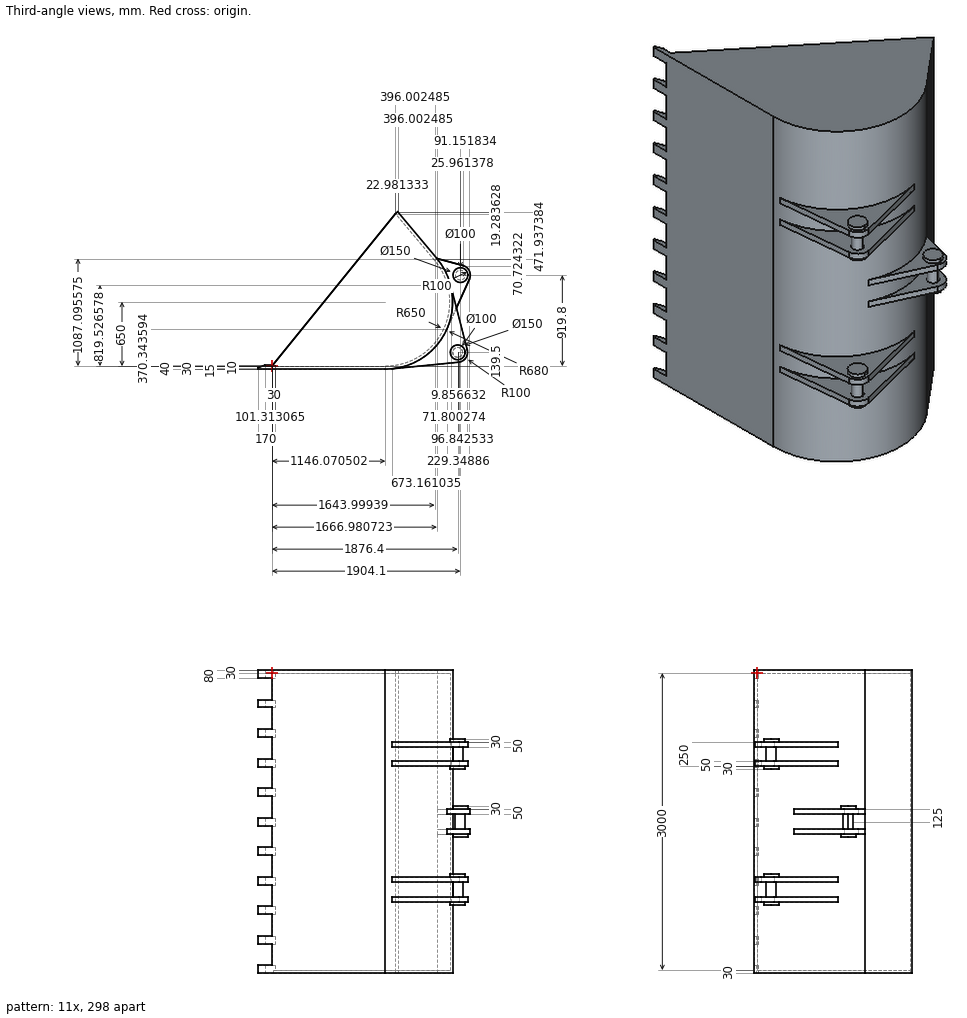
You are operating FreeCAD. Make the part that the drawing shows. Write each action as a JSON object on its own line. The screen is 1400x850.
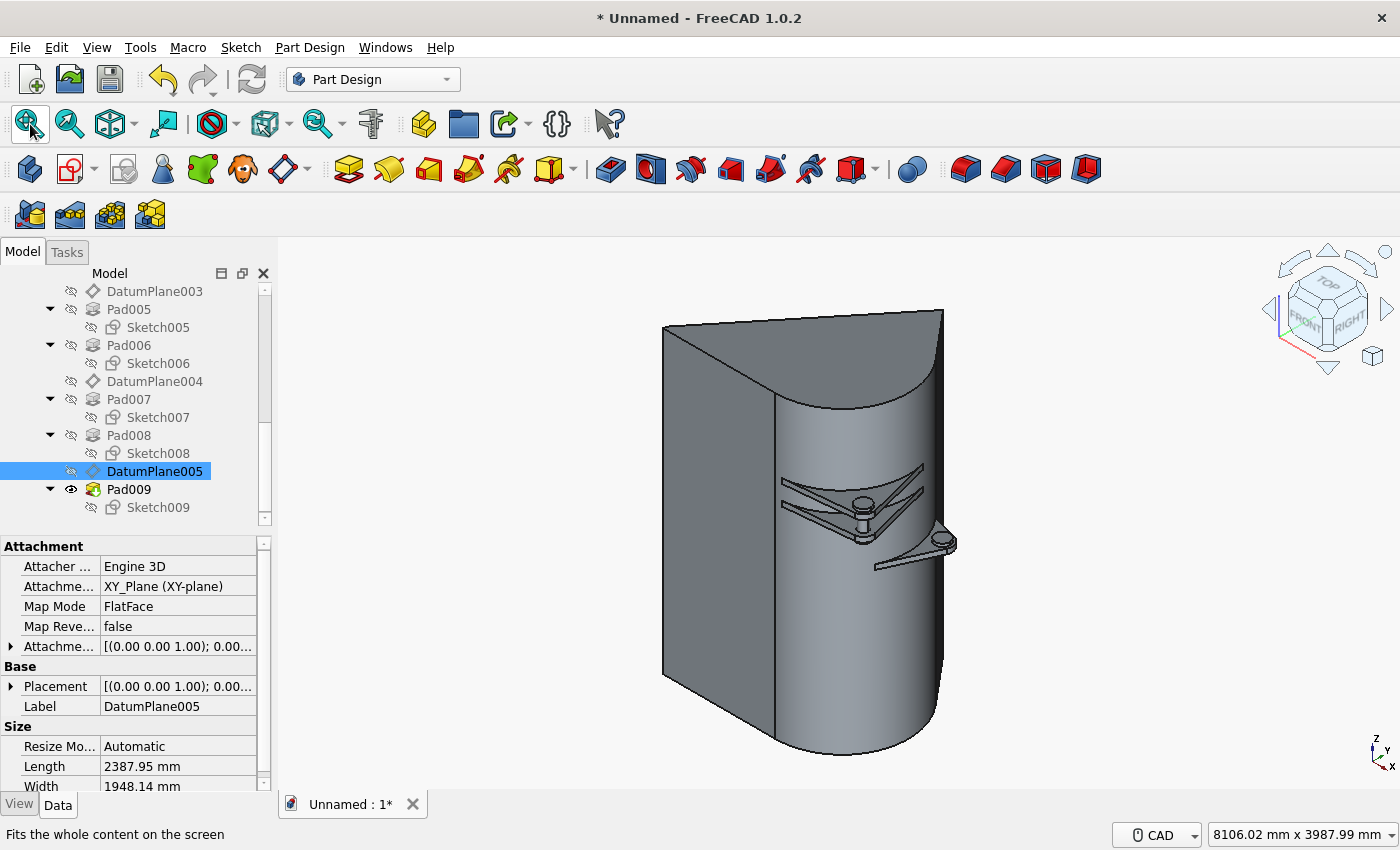
{"action": "scroll", "coordinate": [922, 550], "scroll_direction": "up", "scroll_amount": 4}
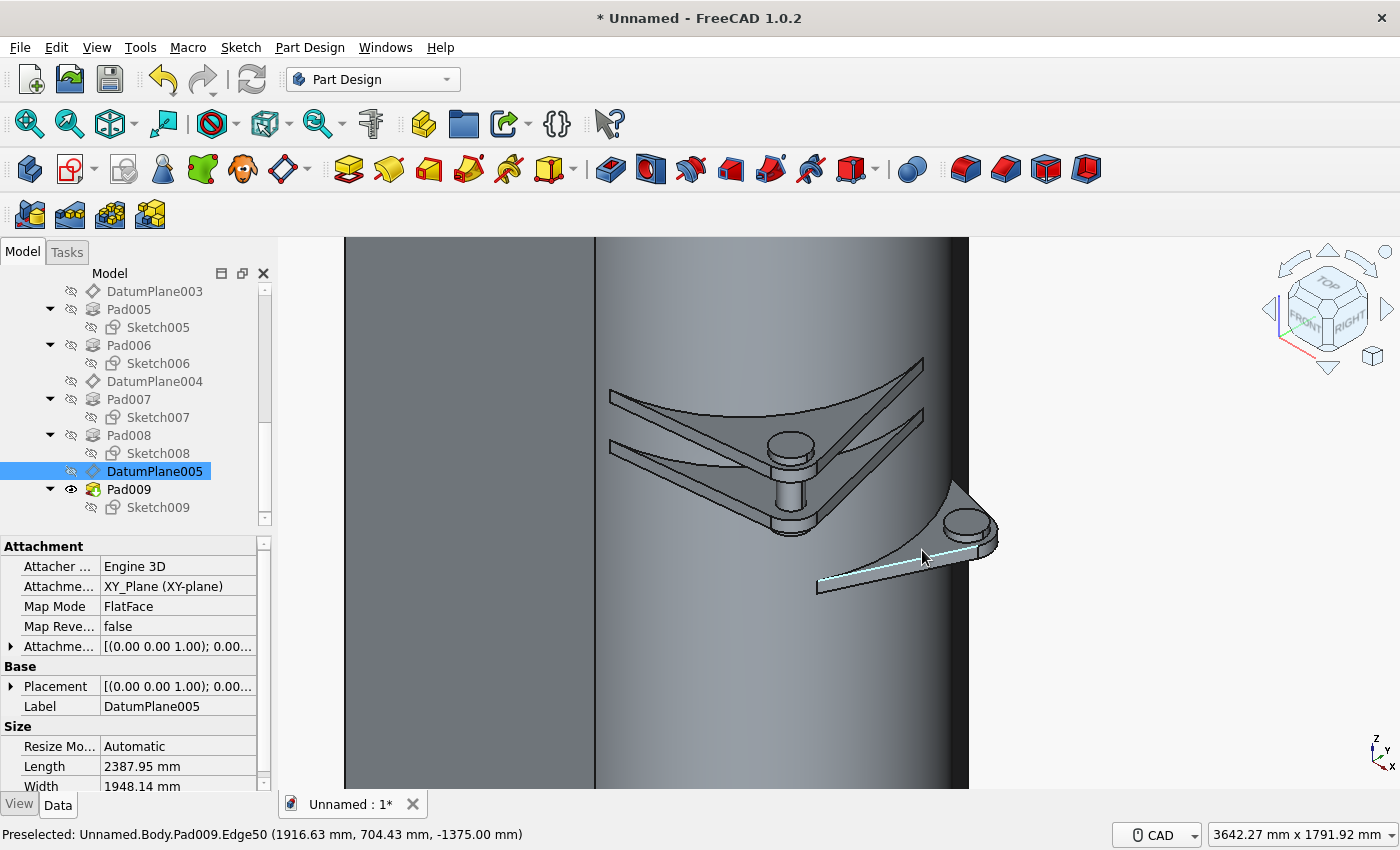
{"action": "left_click", "coordinate": [933, 531]}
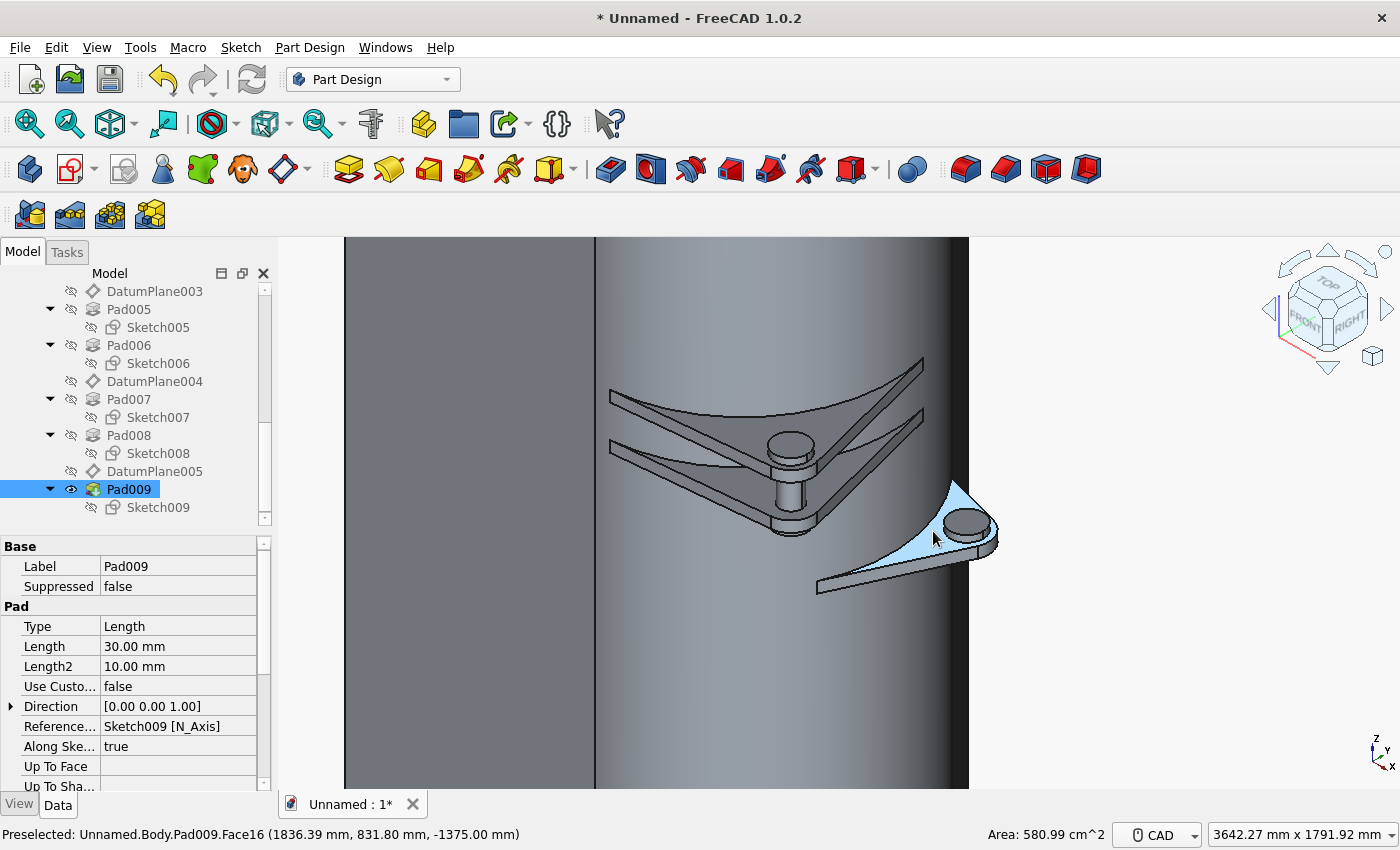
{"action": "left_click", "coordinate": [70, 170]}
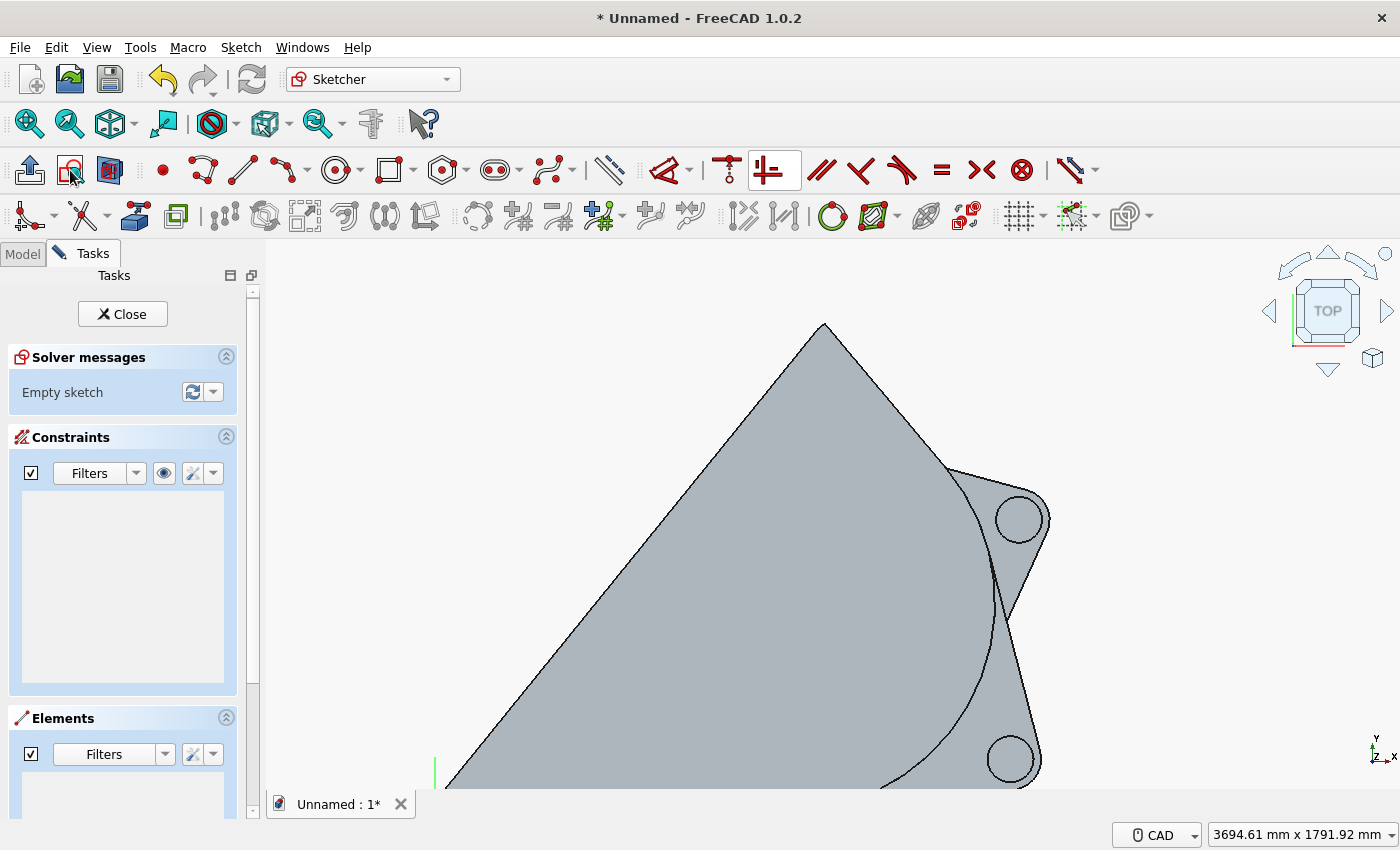
{"action": "scroll", "coordinate": [1044, 520], "scroll_direction": "up", "scroll_amount": 12}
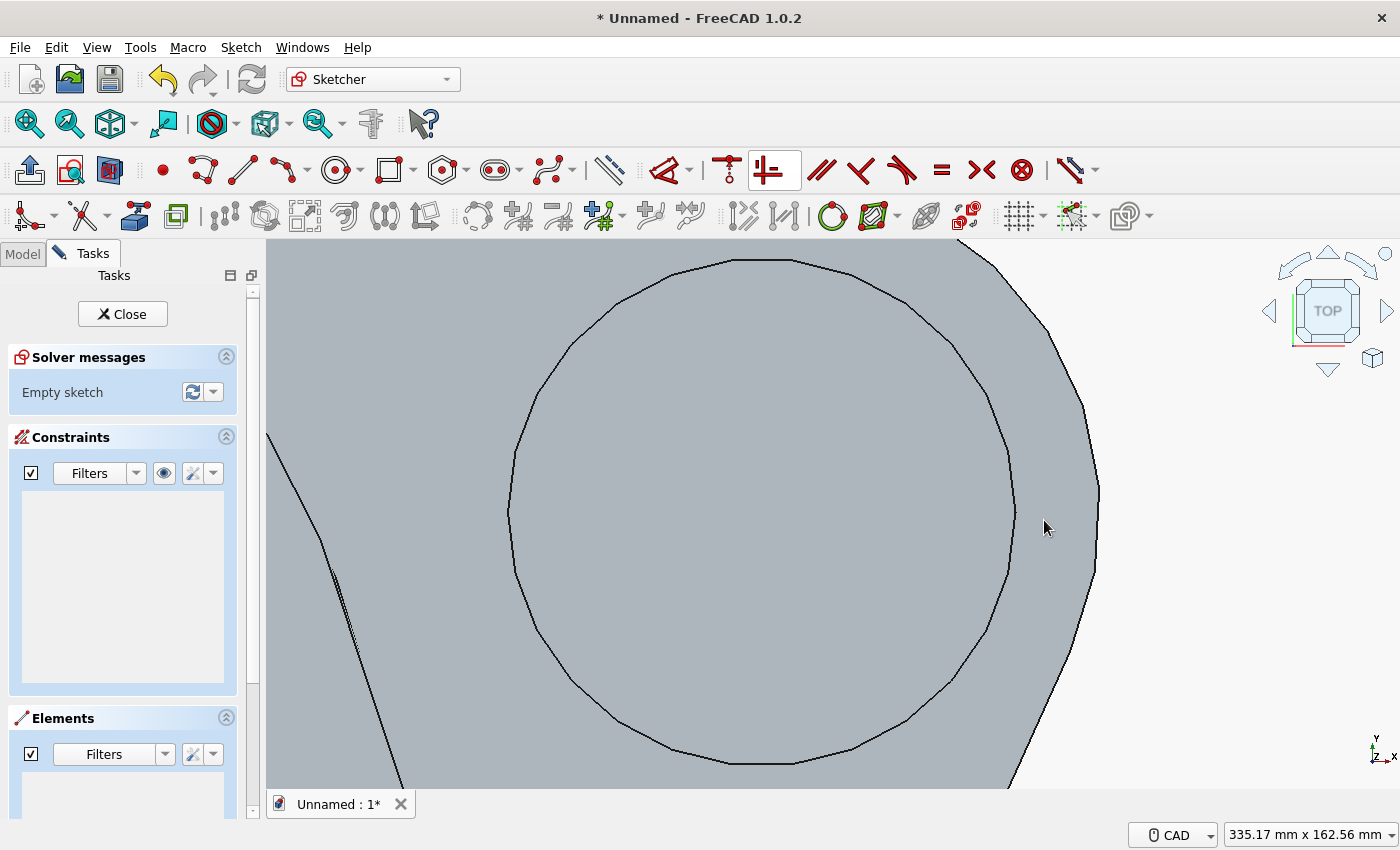
{"action": "left_click", "coordinate": [336, 170]}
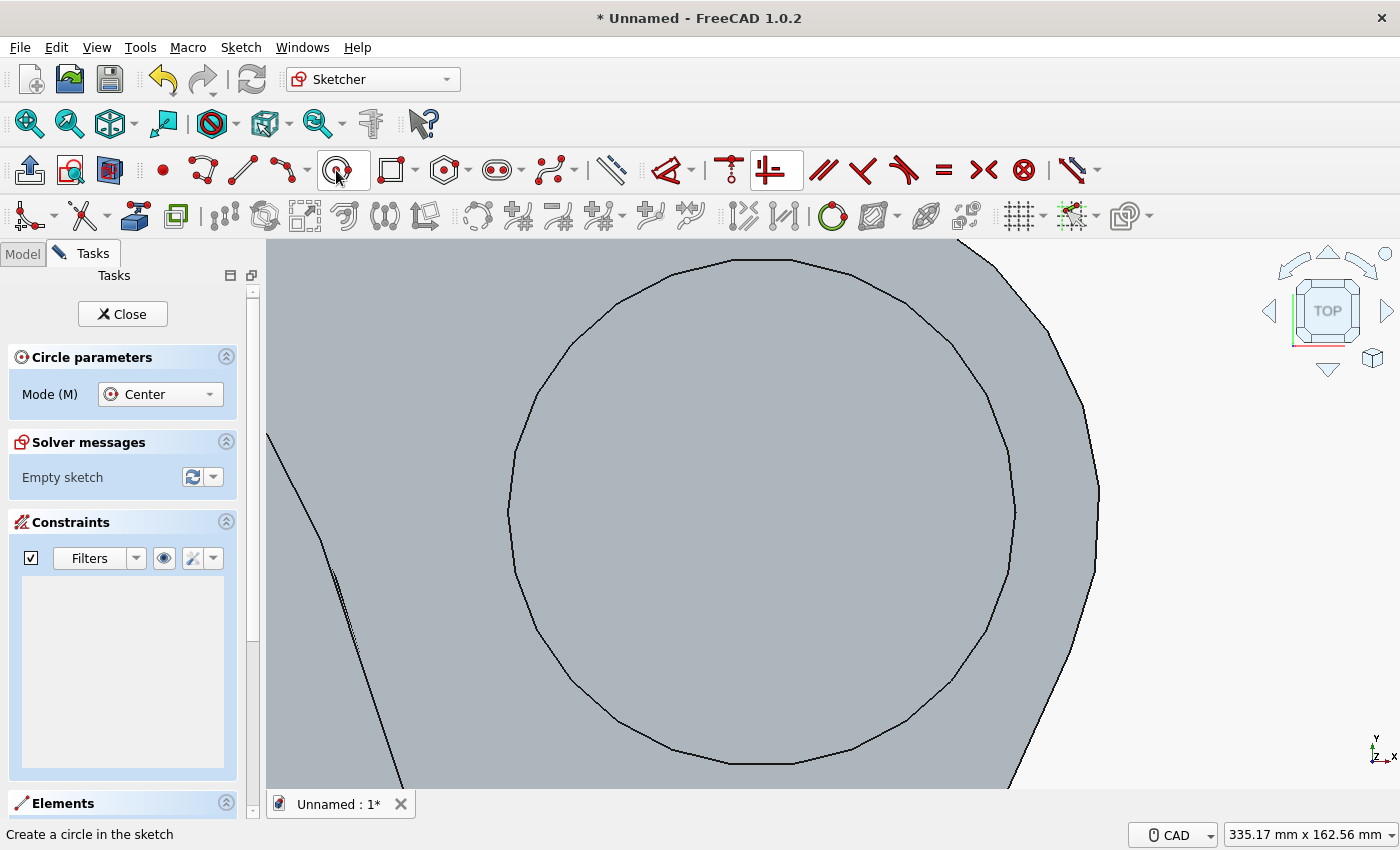
{"action": "left_click", "coordinate": [762, 512]}
{"action": "left_click", "coordinate": [881, 393]}
{"action": "key", "text": "Escape"}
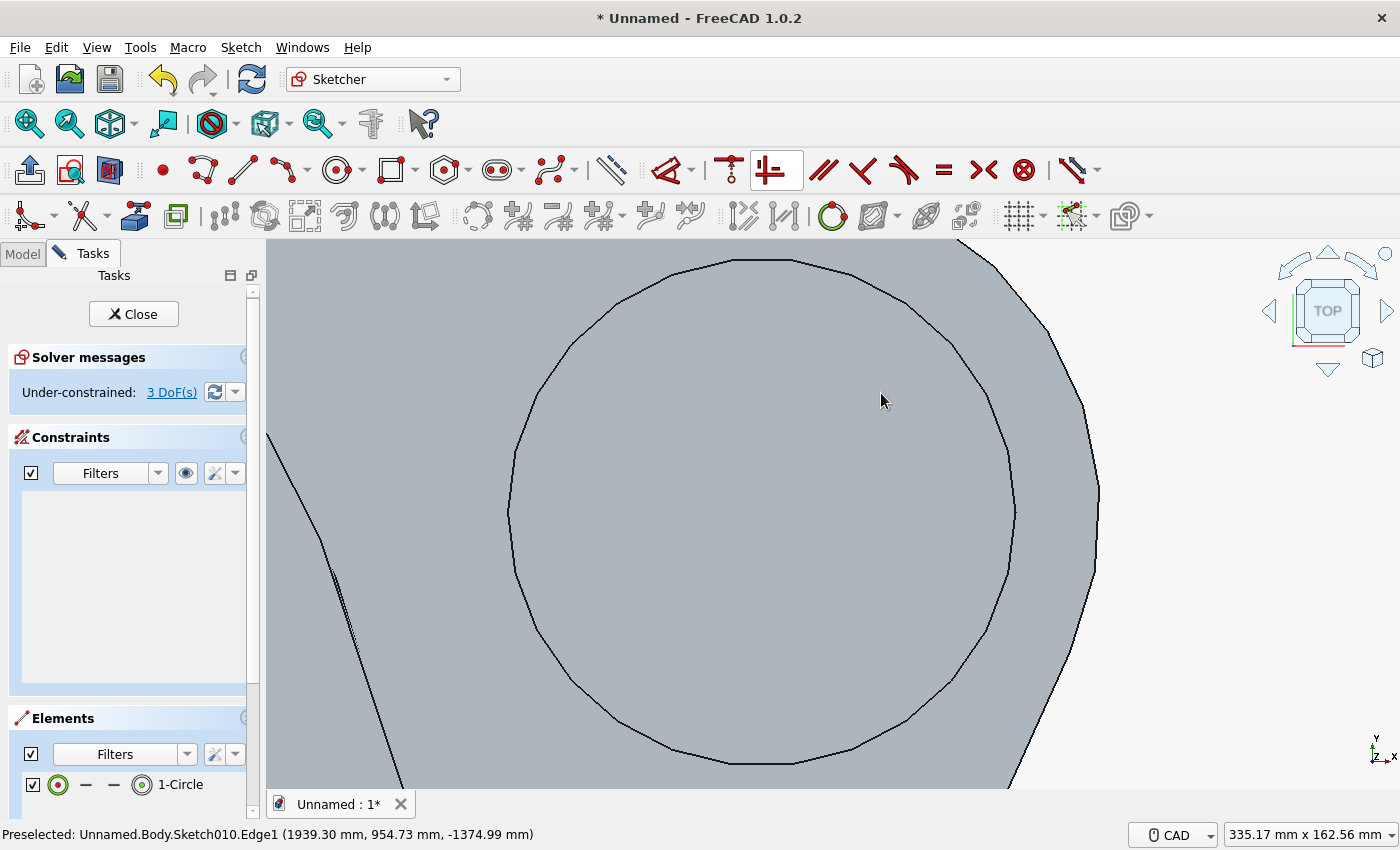
{"action": "left_click", "coordinate": [666, 170]}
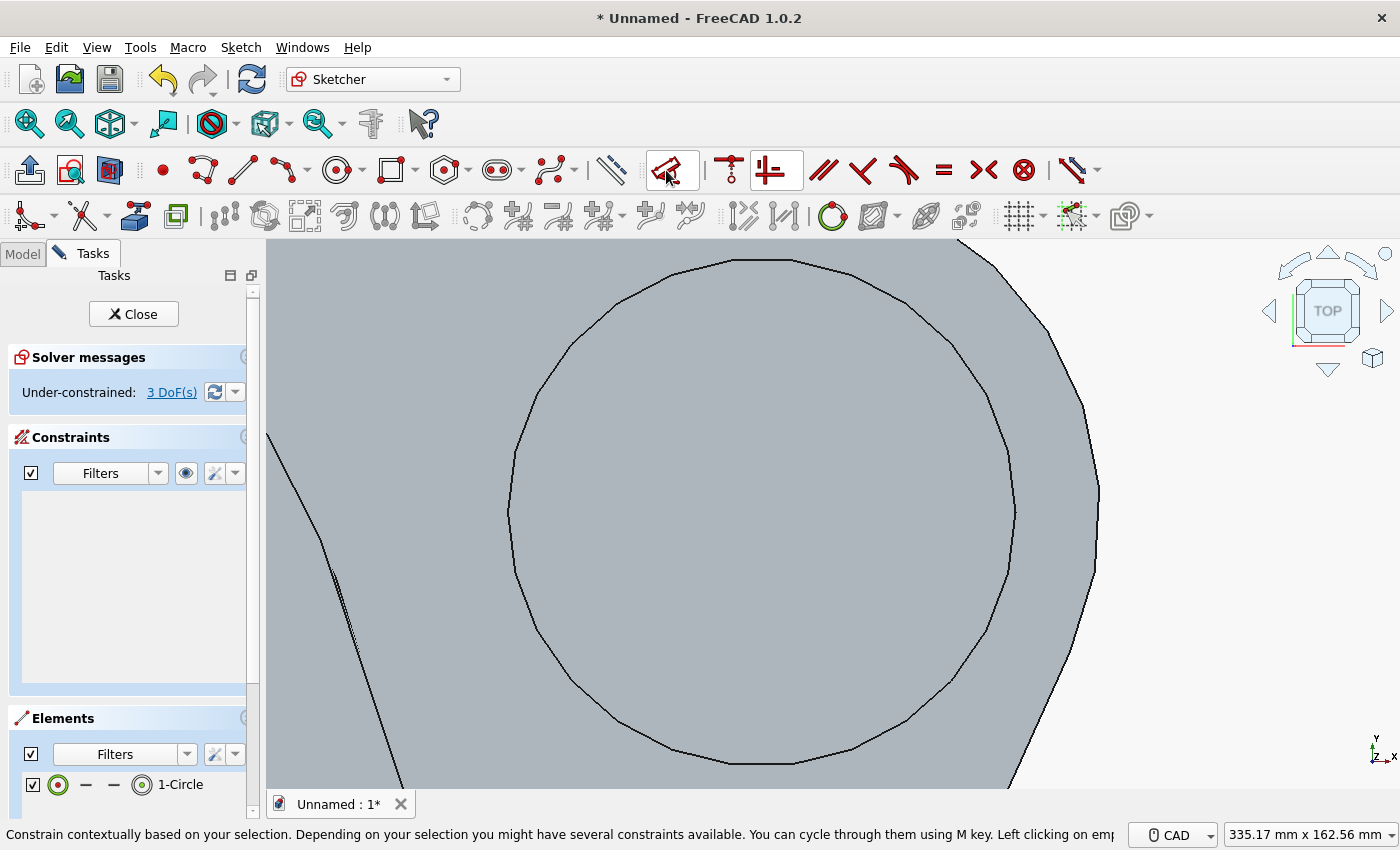
{"action": "left_click", "coordinate": [881, 394]}
{"action": "left_click", "coordinate": [904, 371]}